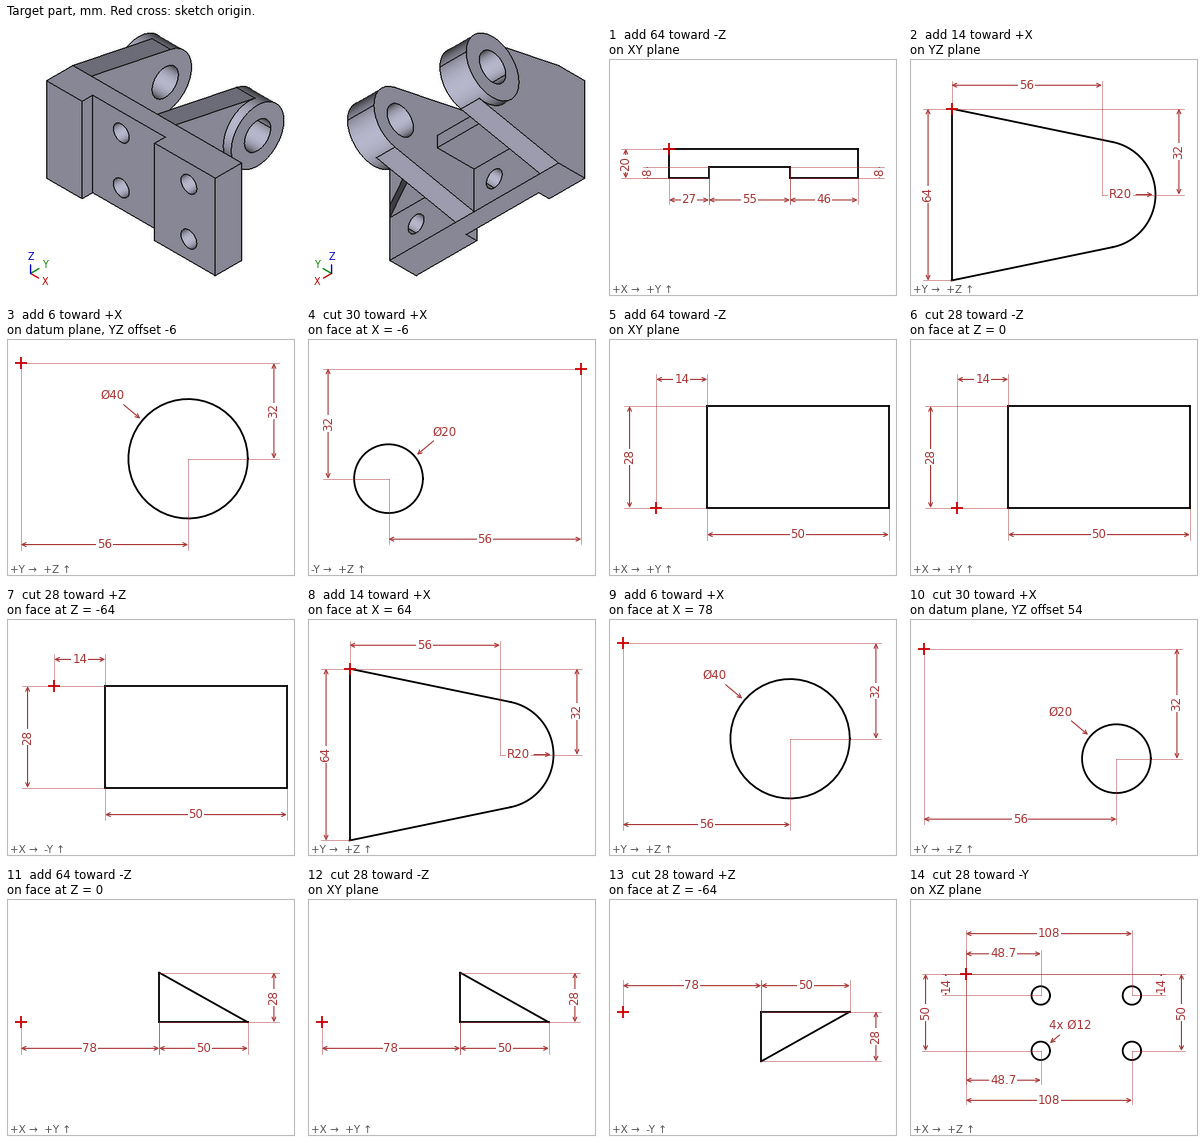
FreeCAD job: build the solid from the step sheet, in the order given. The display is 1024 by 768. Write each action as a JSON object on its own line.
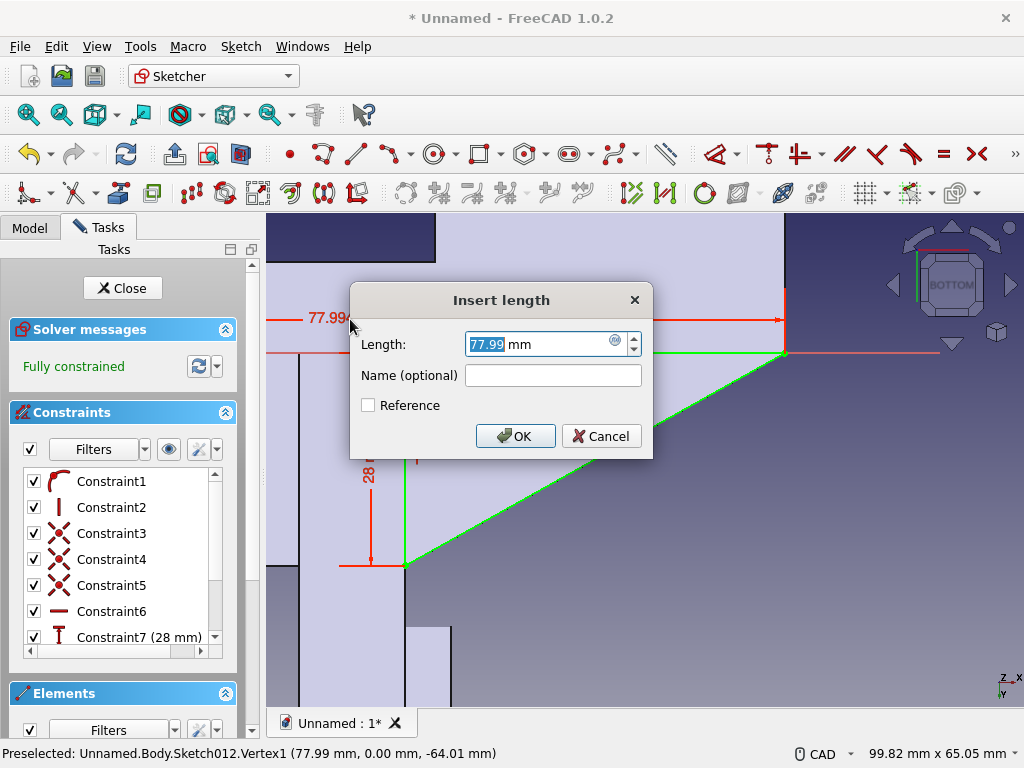
{"action": "type", "text": "78"}
{"action": "key", "text": "Return"}
{"action": "key", "text": "Escape"}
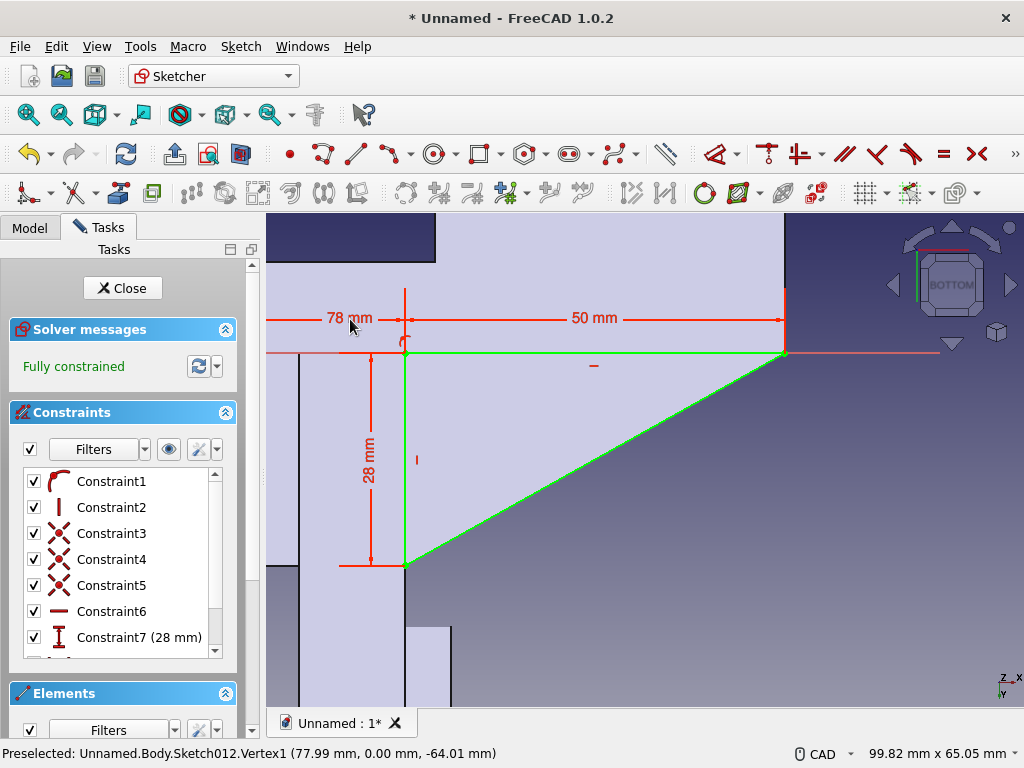
{"action": "left_click", "coordinate": [123, 288]}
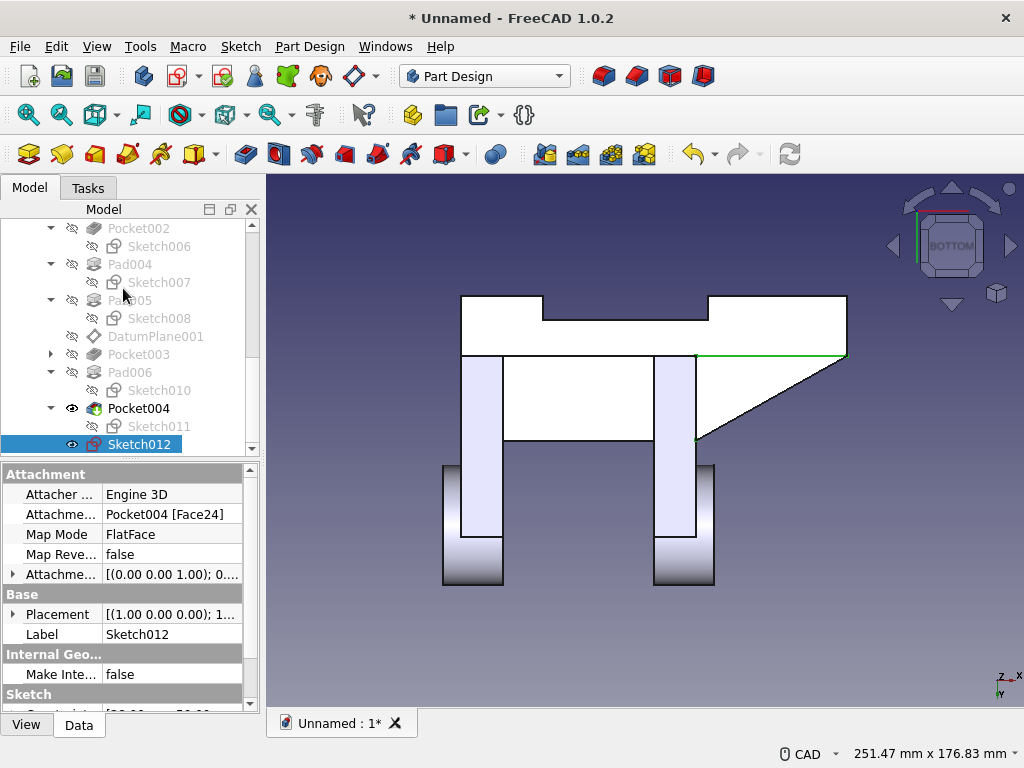
{"action": "left_click", "coordinate": [246, 154]}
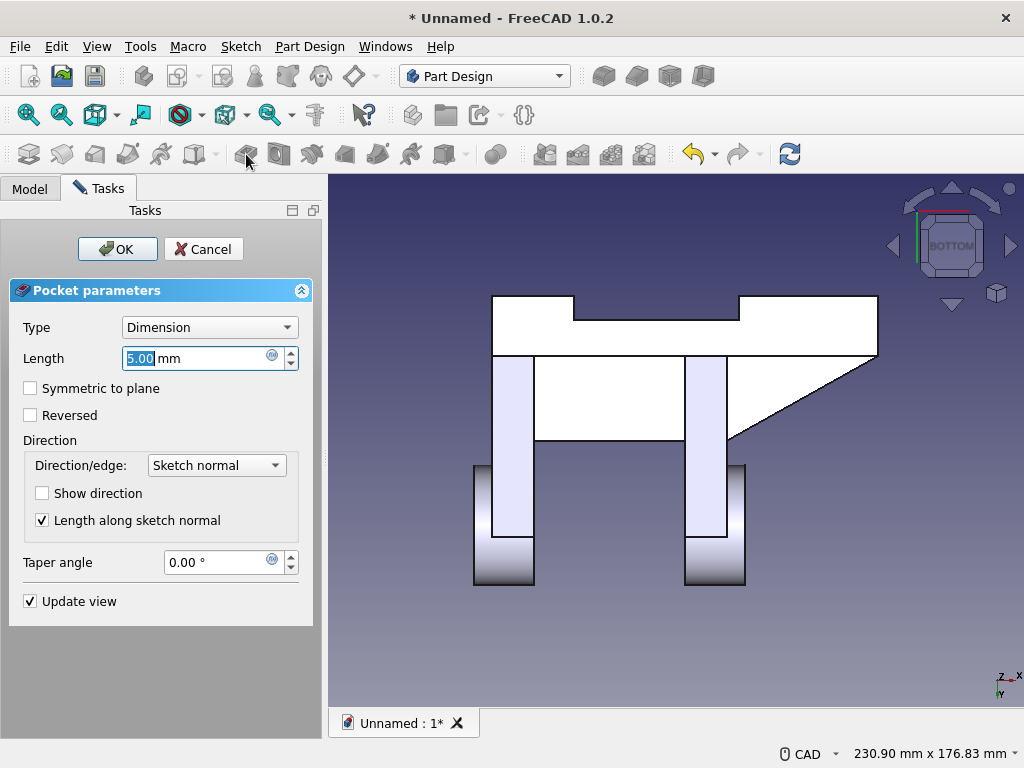
{"action": "type", "text": "28"}
{"action": "key", "text": "Tab"}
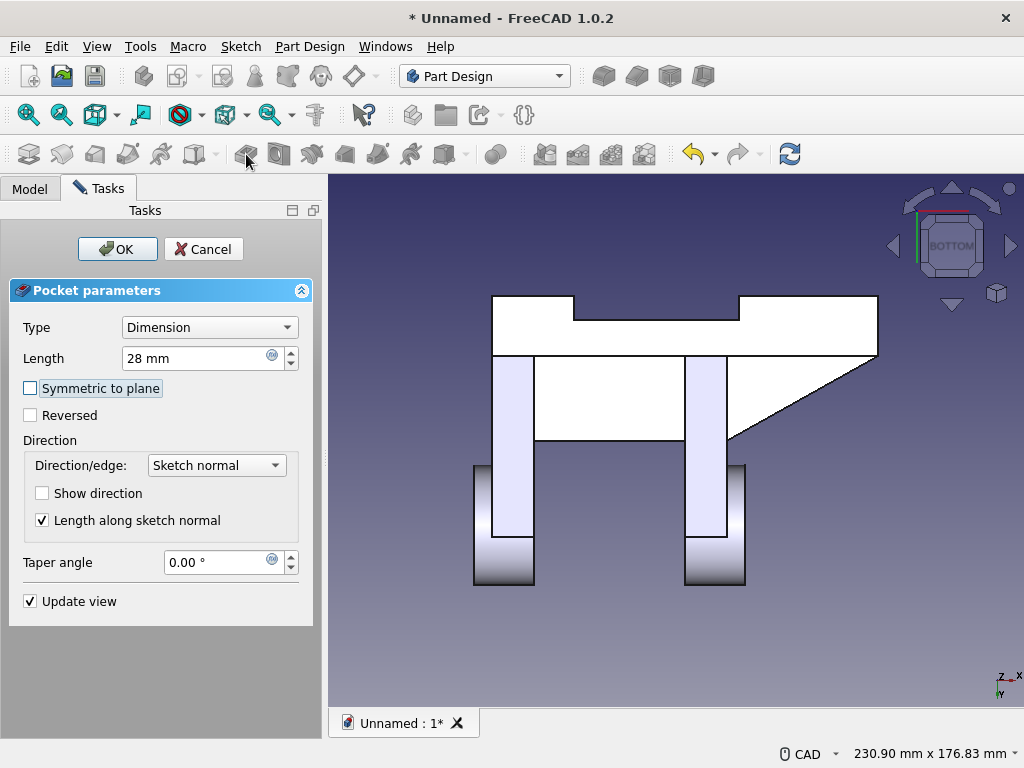
{"action": "left_click", "coordinate": [118, 249]}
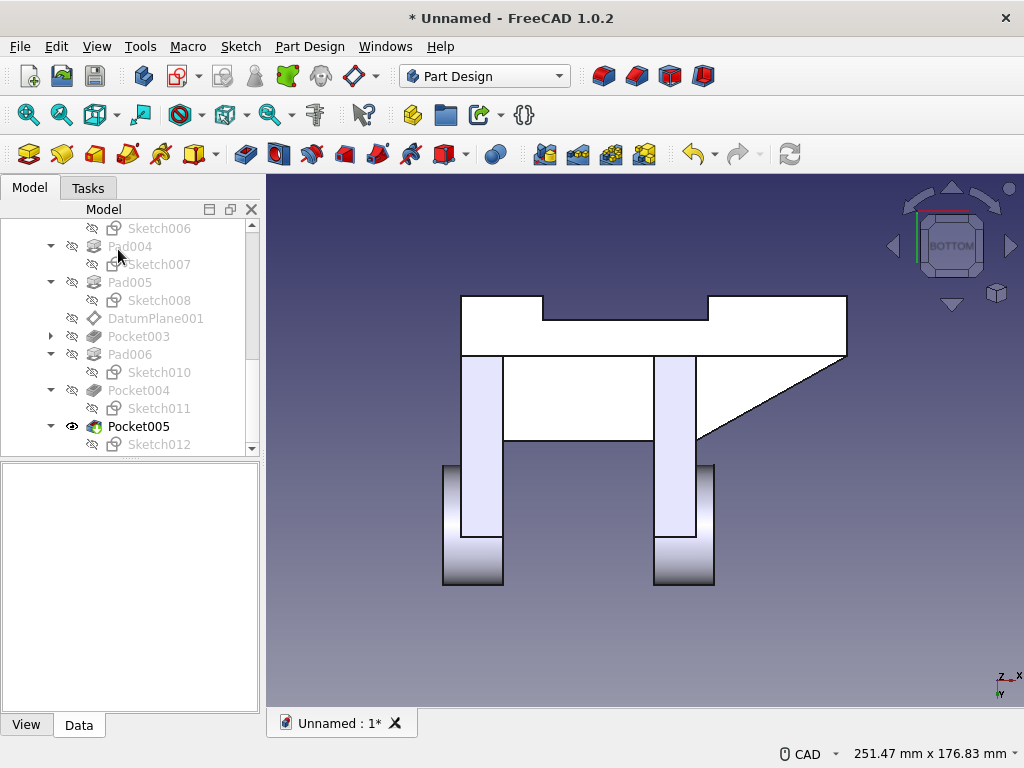
{"action": "left_click", "coordinate": [176, 76]}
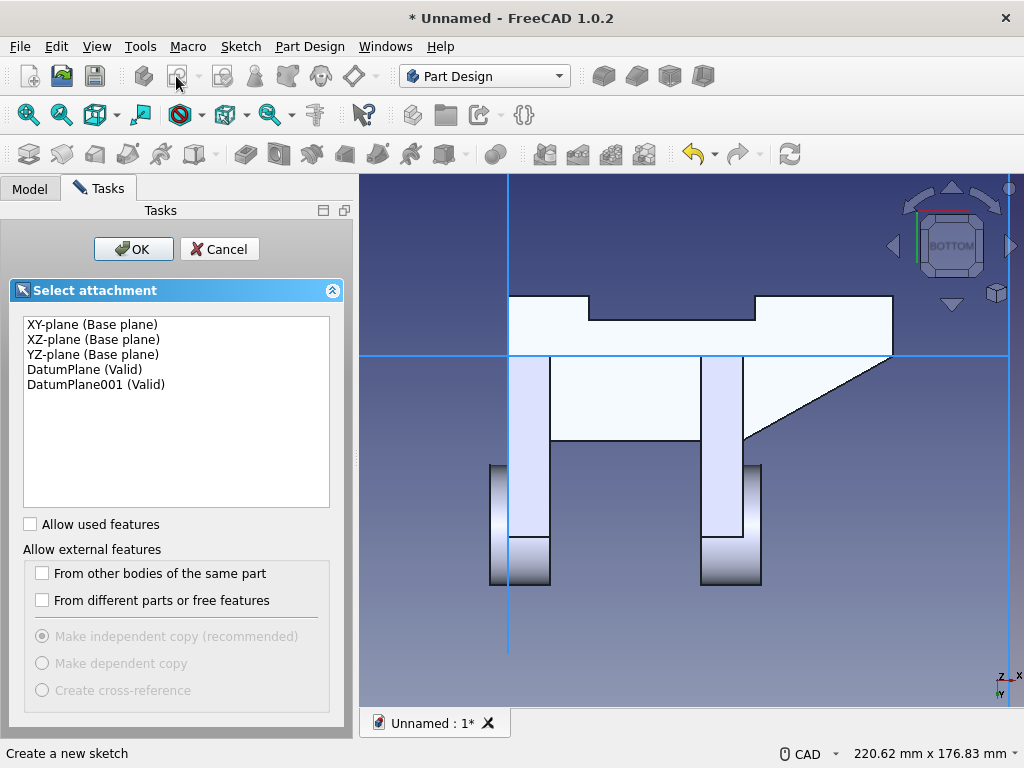
{"action": "left_click", "coordinate": [84, 340]}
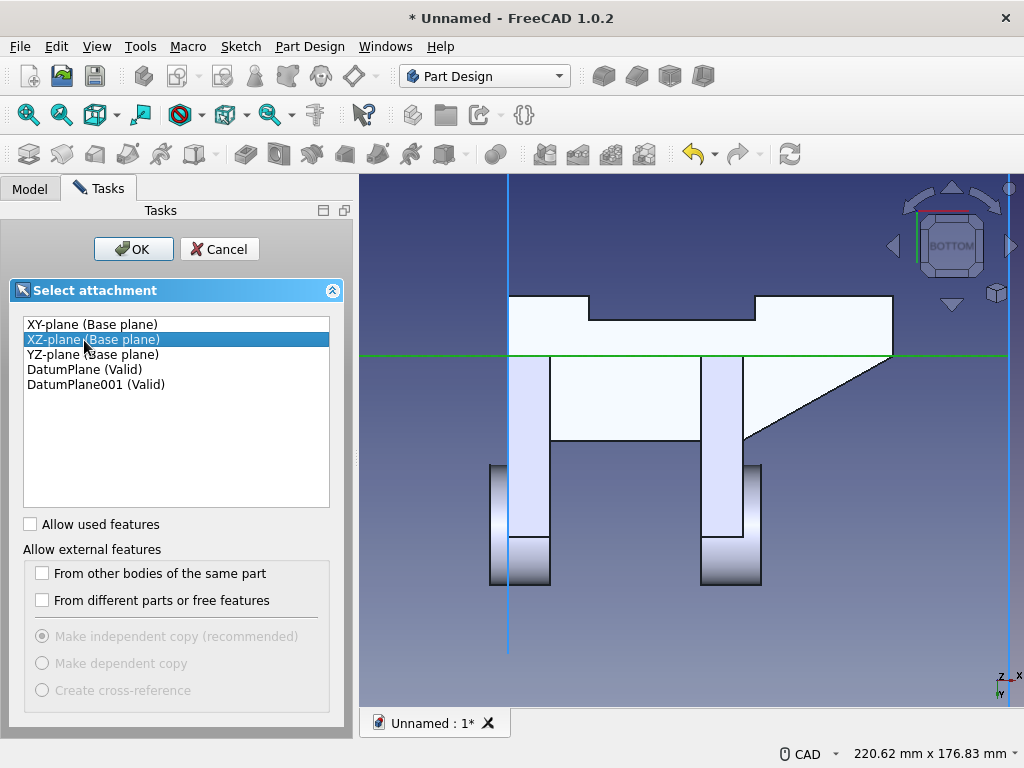
{"action": "left_click", "coordinate": [134, 249]}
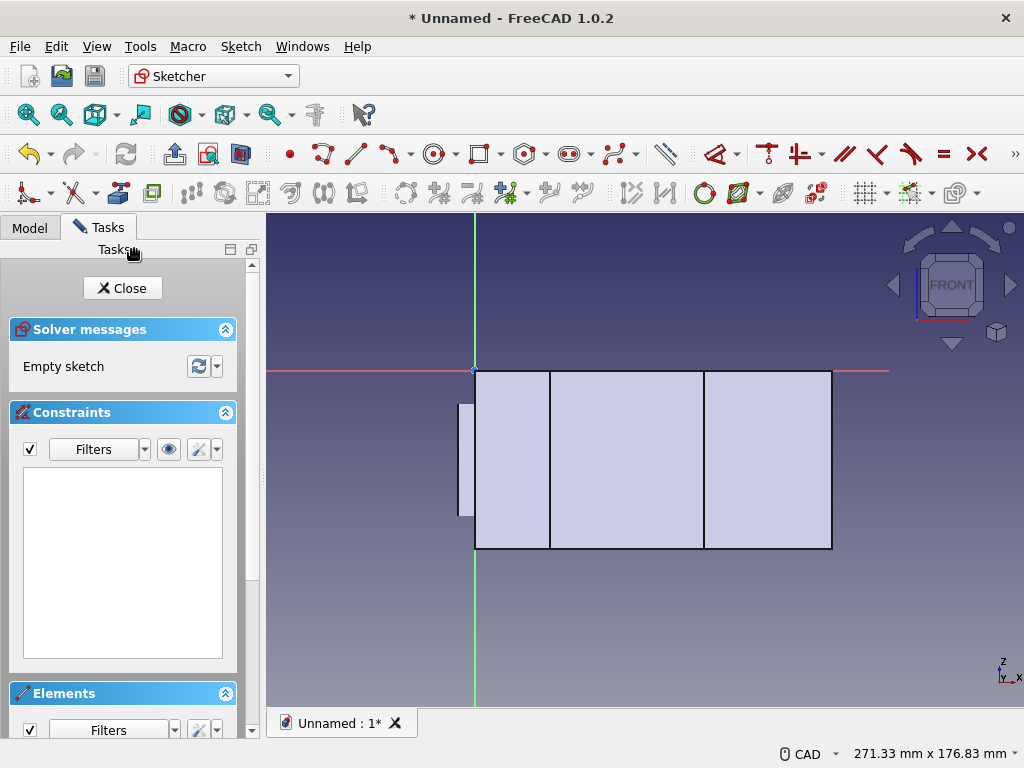
{"action": "left_click", "coordinate": [241, 154]}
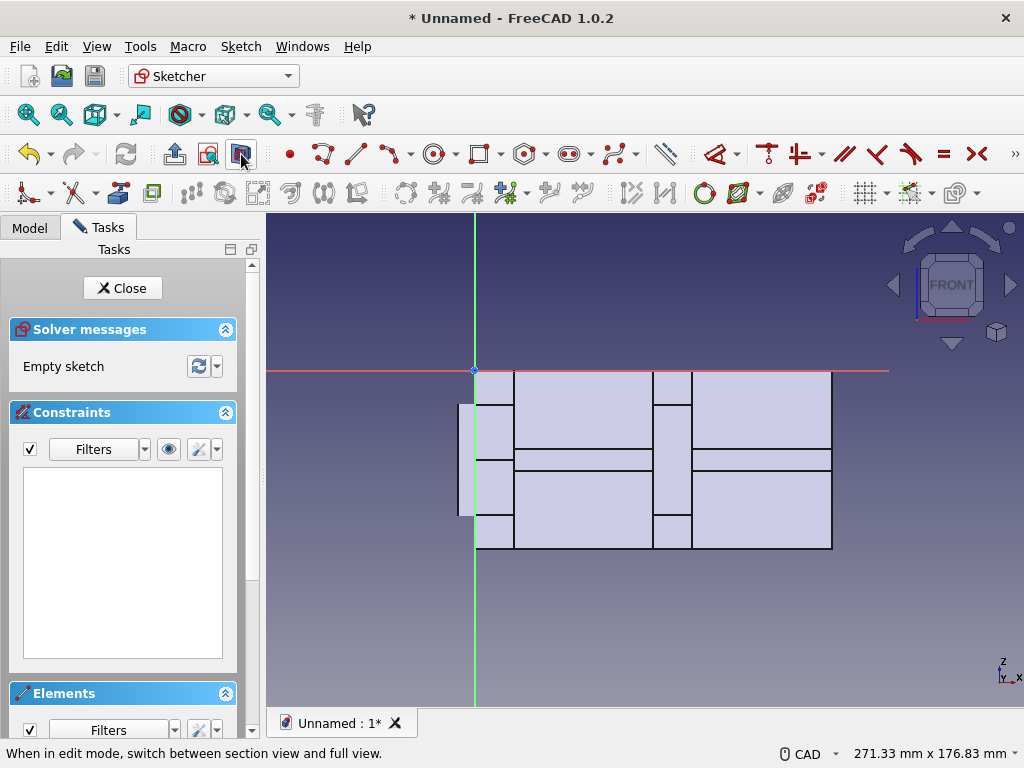
{"action": "left_click", "coordinate": [434, 154]}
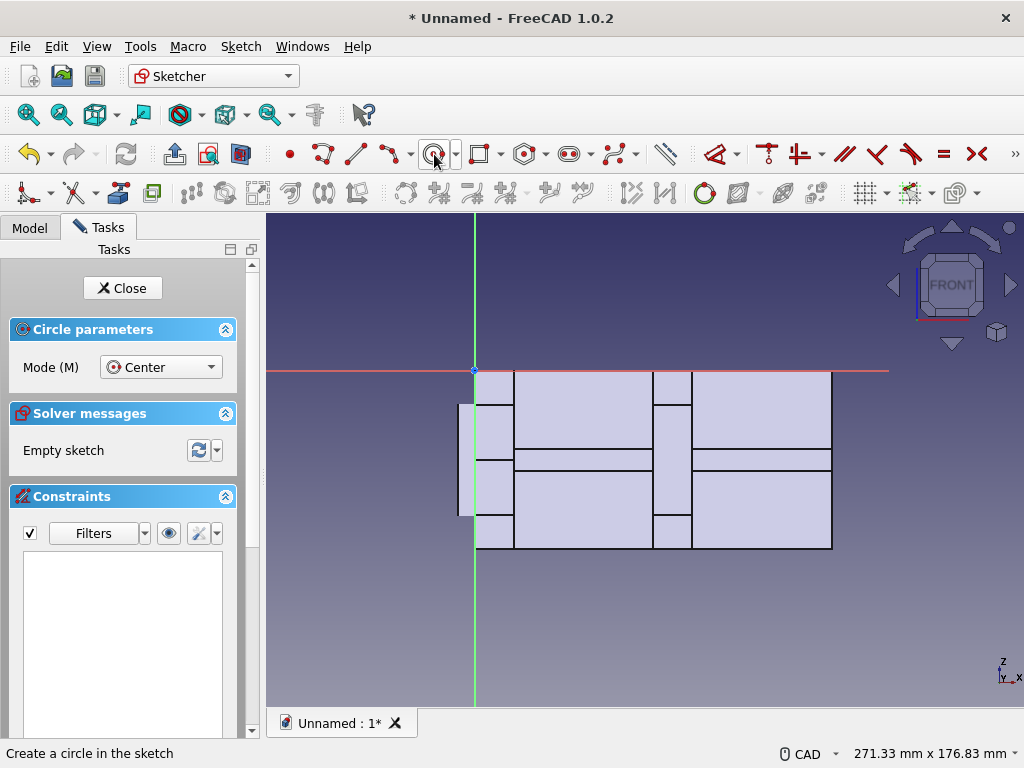
{"action": "scroll", "coordinate": [611, 510], "scroll_direction": "up", "scroll_amount": 2}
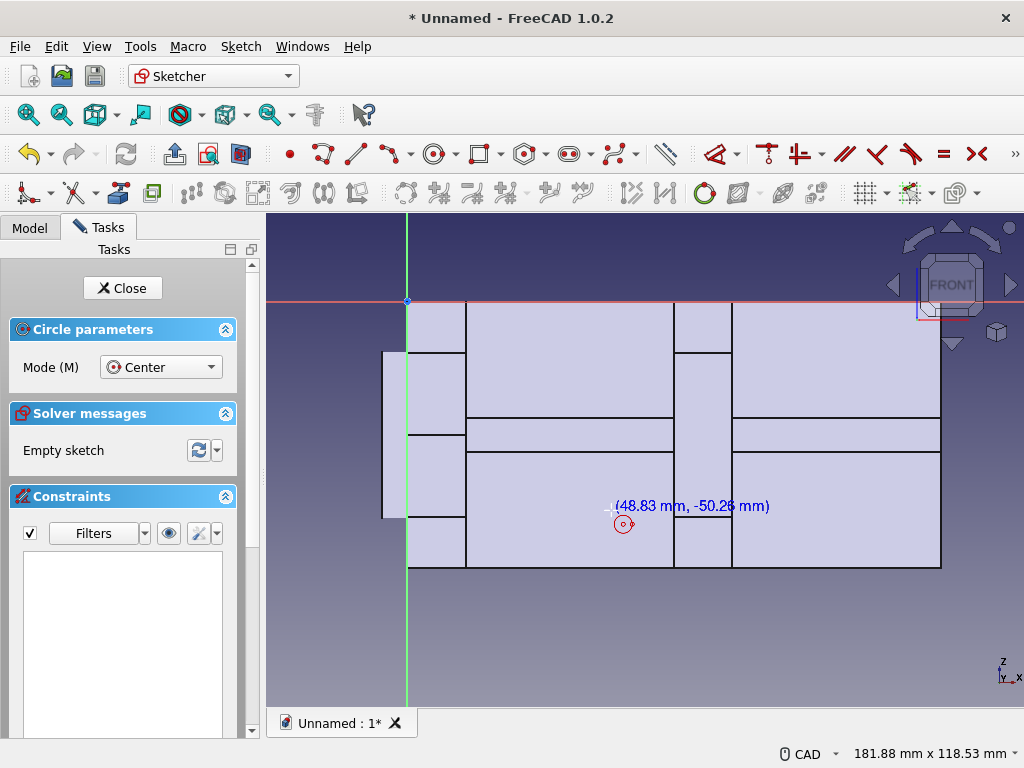
{"action": "left_click", "coordinate": [610, 510]}
{"action": "left_click", "coordinate": [628, 492]}